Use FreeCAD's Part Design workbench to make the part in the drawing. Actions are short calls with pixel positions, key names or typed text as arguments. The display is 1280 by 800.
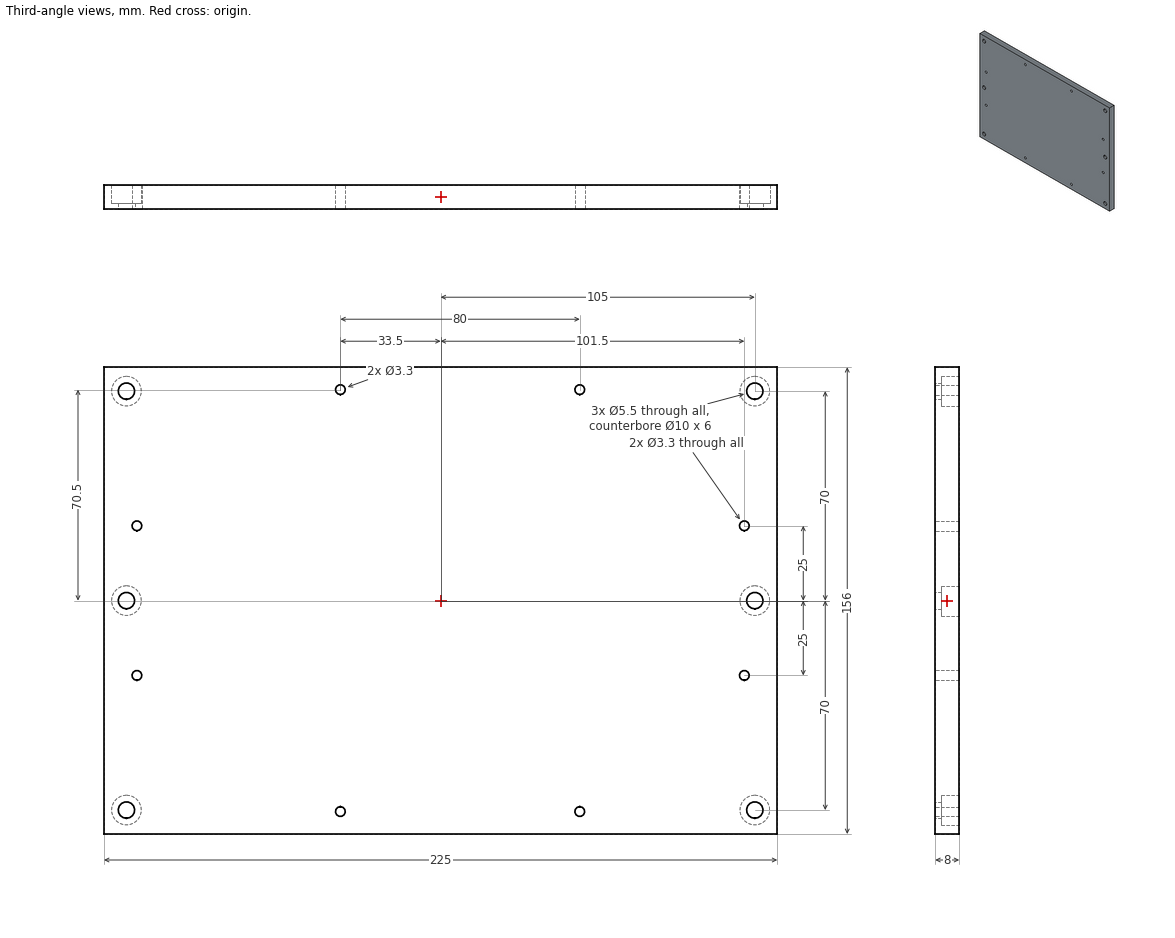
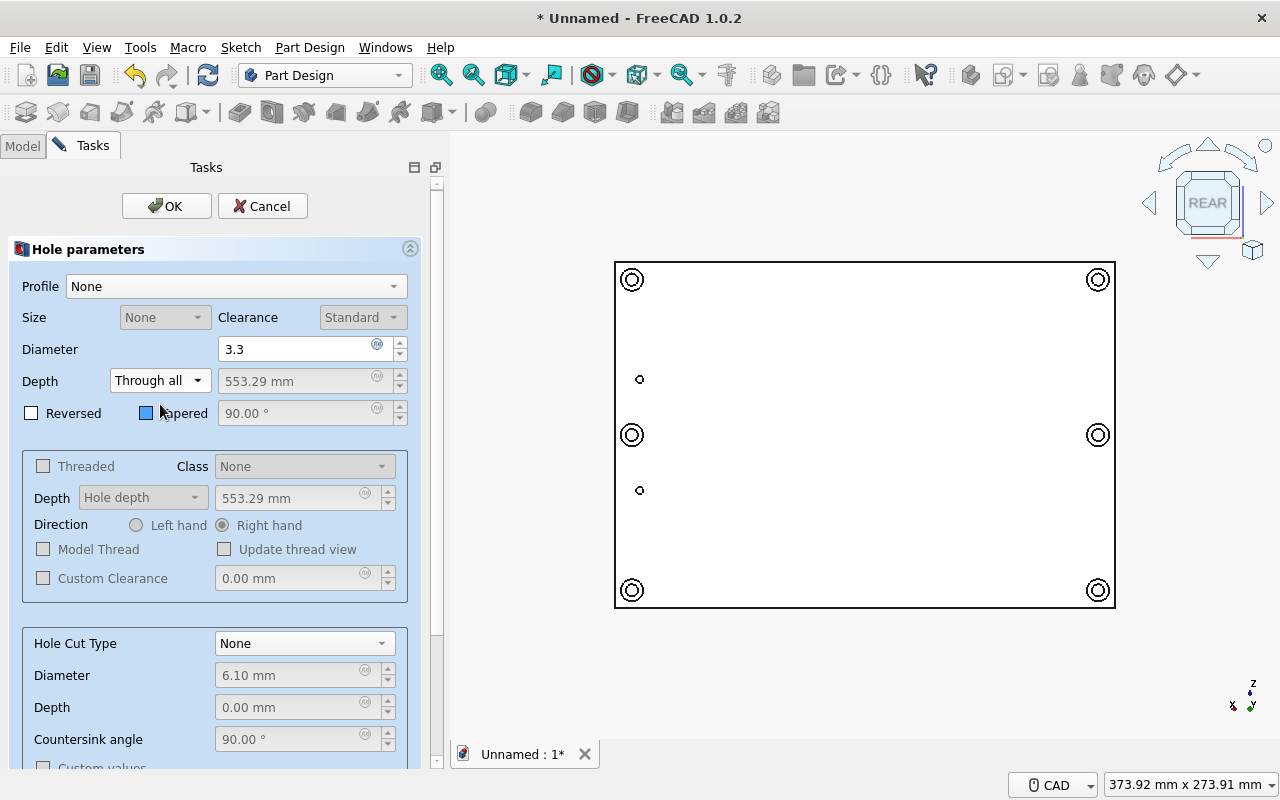
click(167, 206)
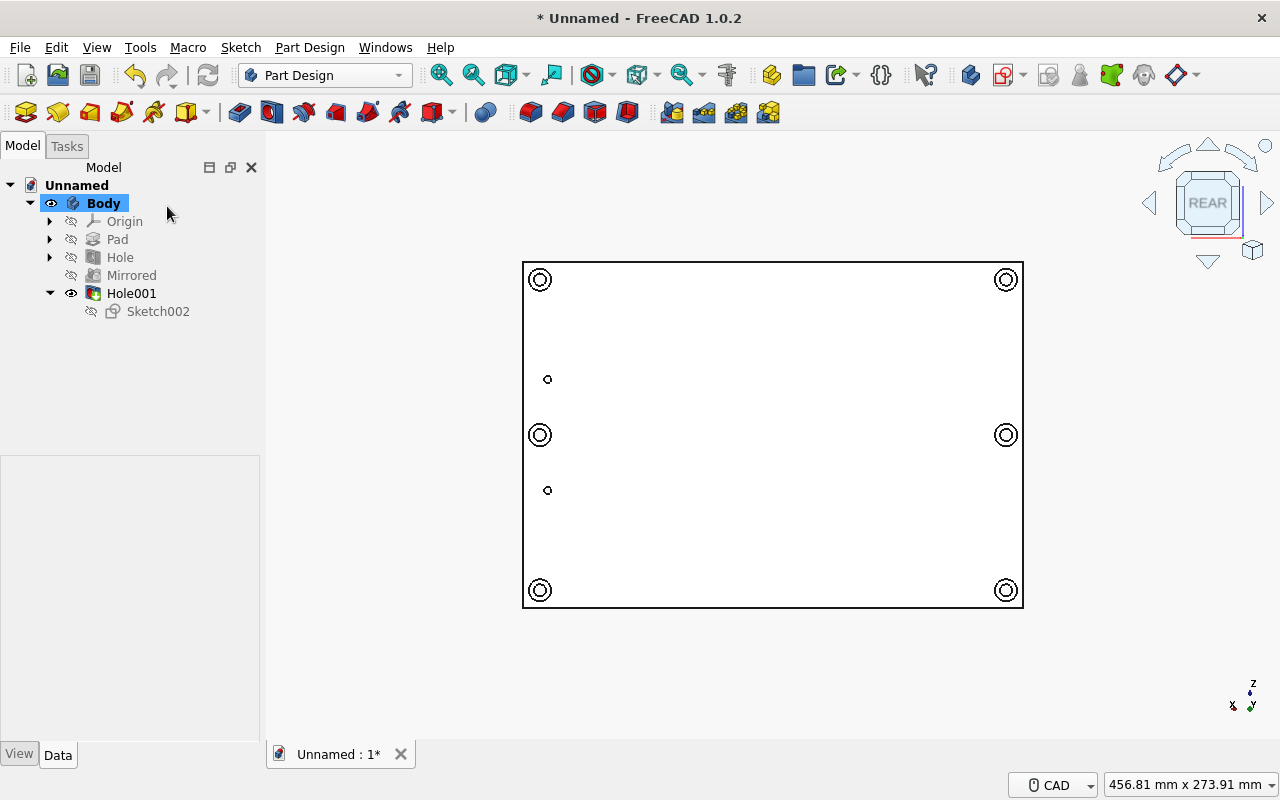
click(773, 434)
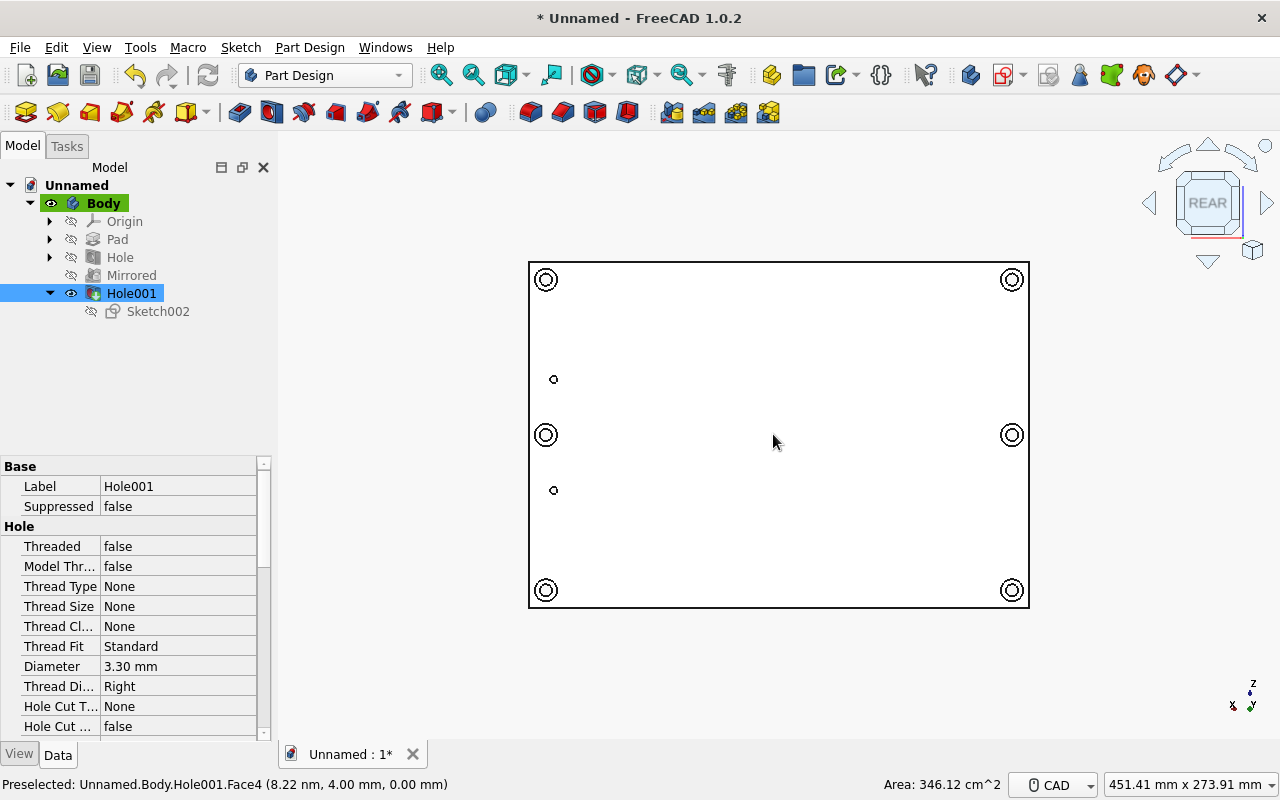
click(1004, 76)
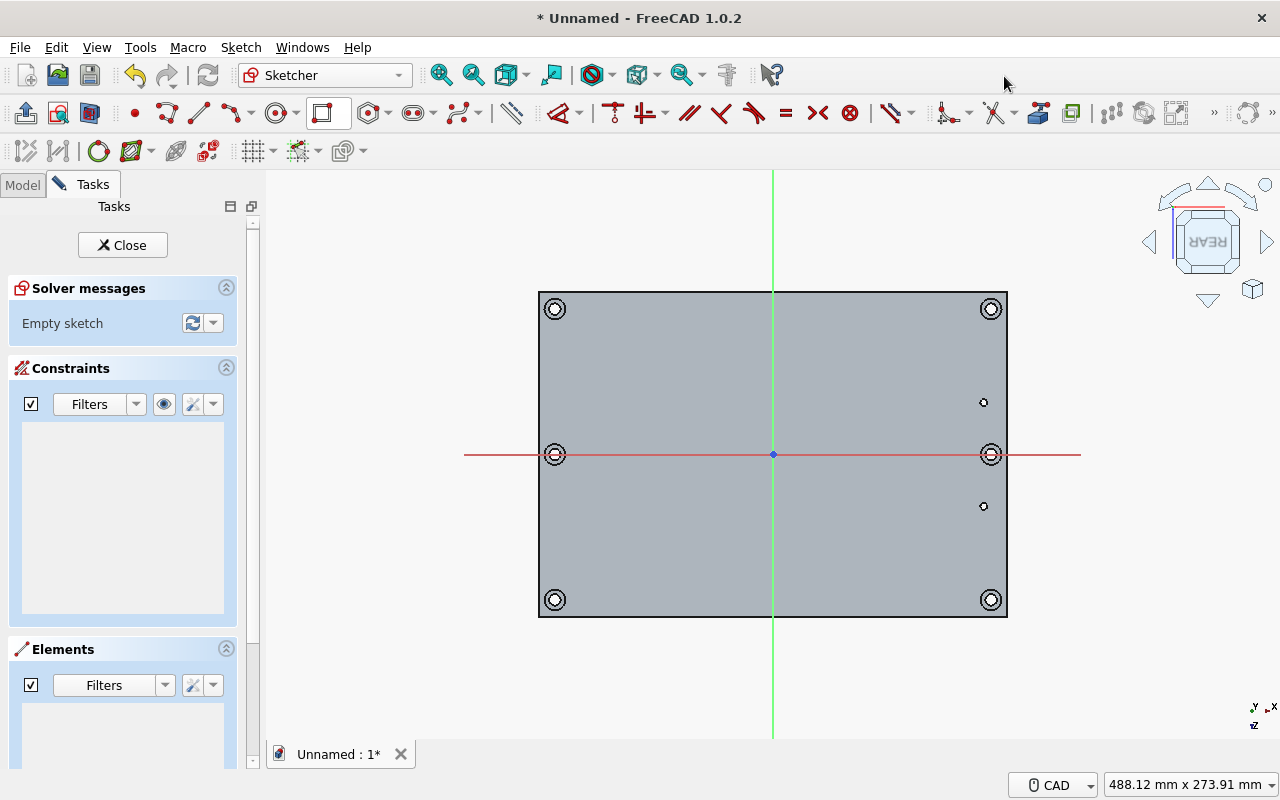
scroll(853, 591, up, 4)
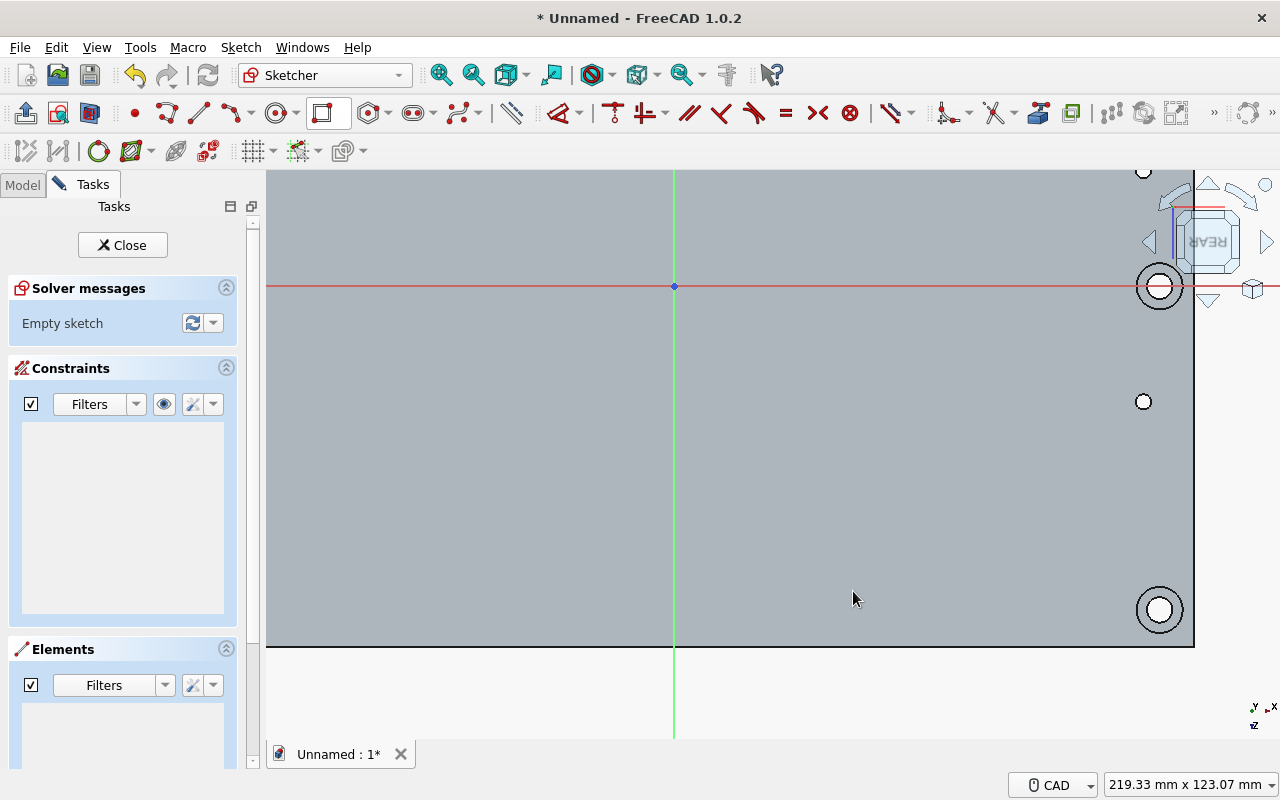
click(276, 114)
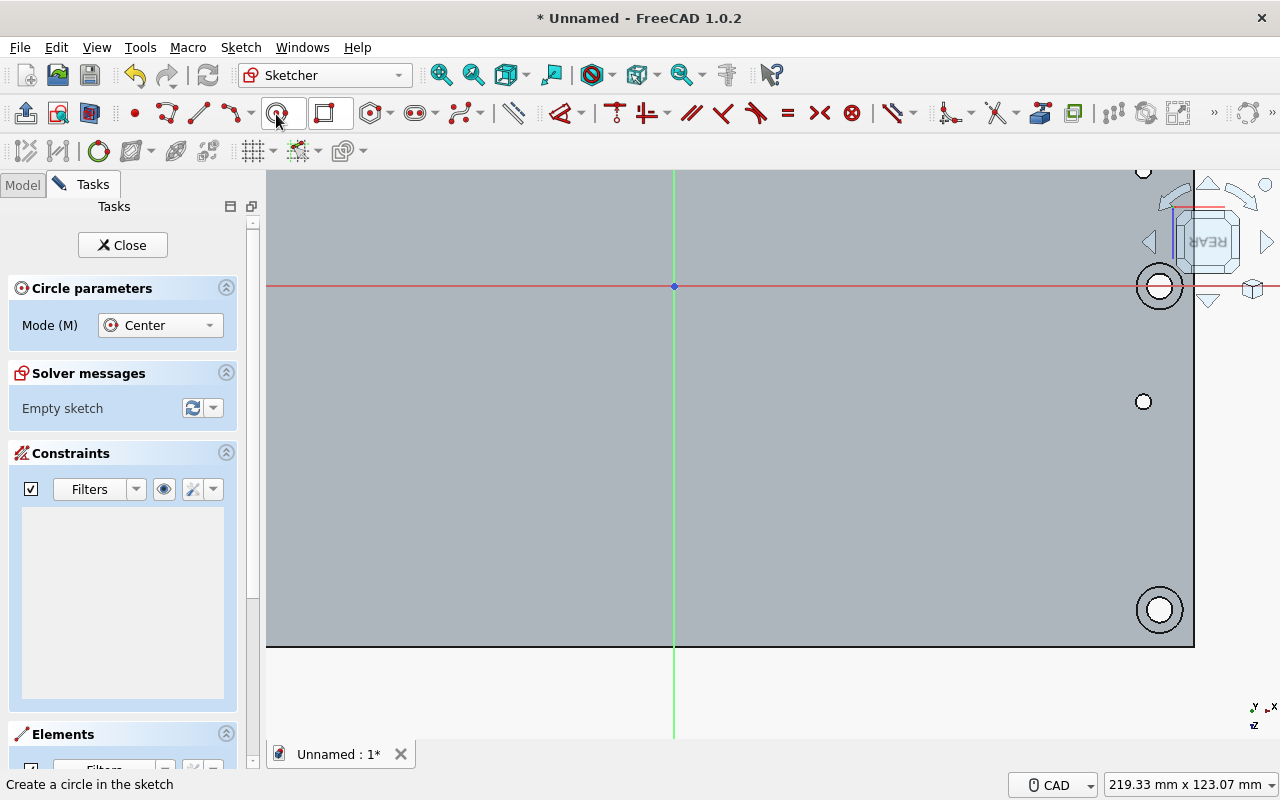
scroll(519, 612, up, 6)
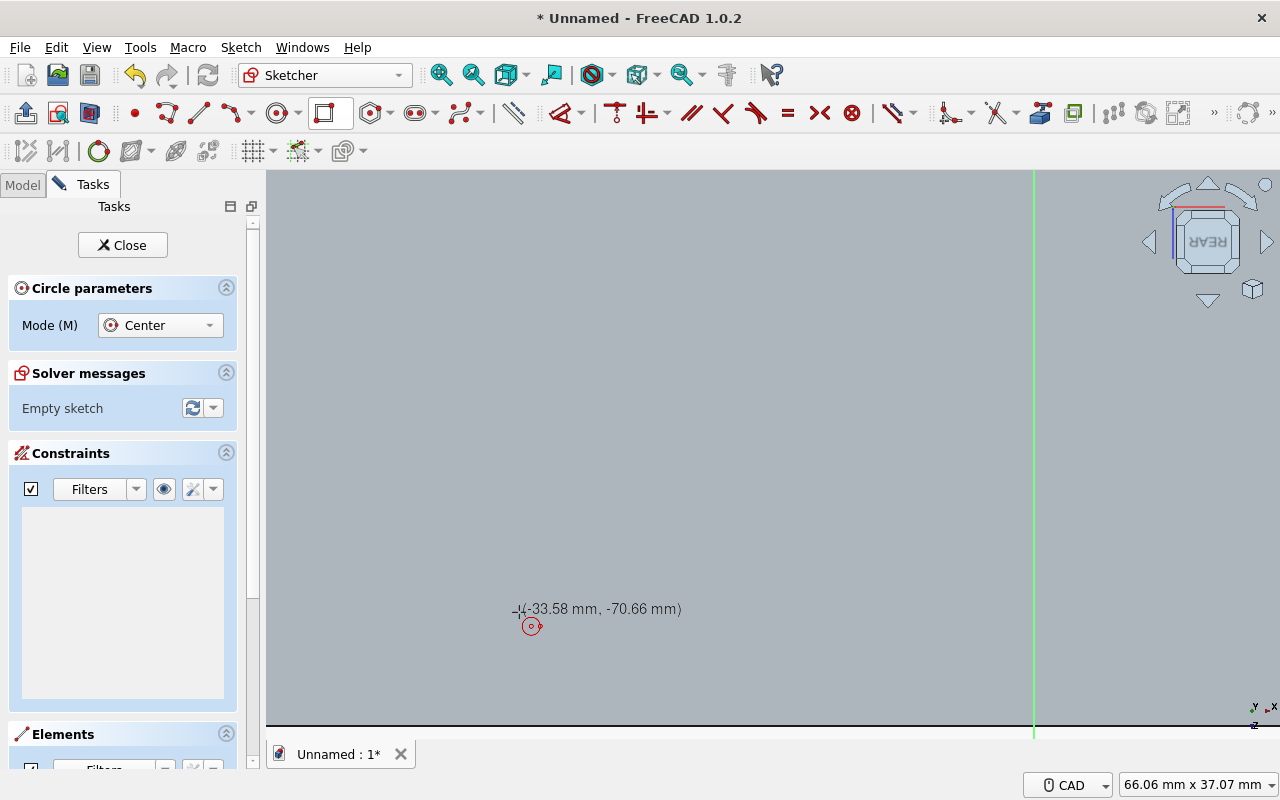
click(520, 611)
click(538, 593)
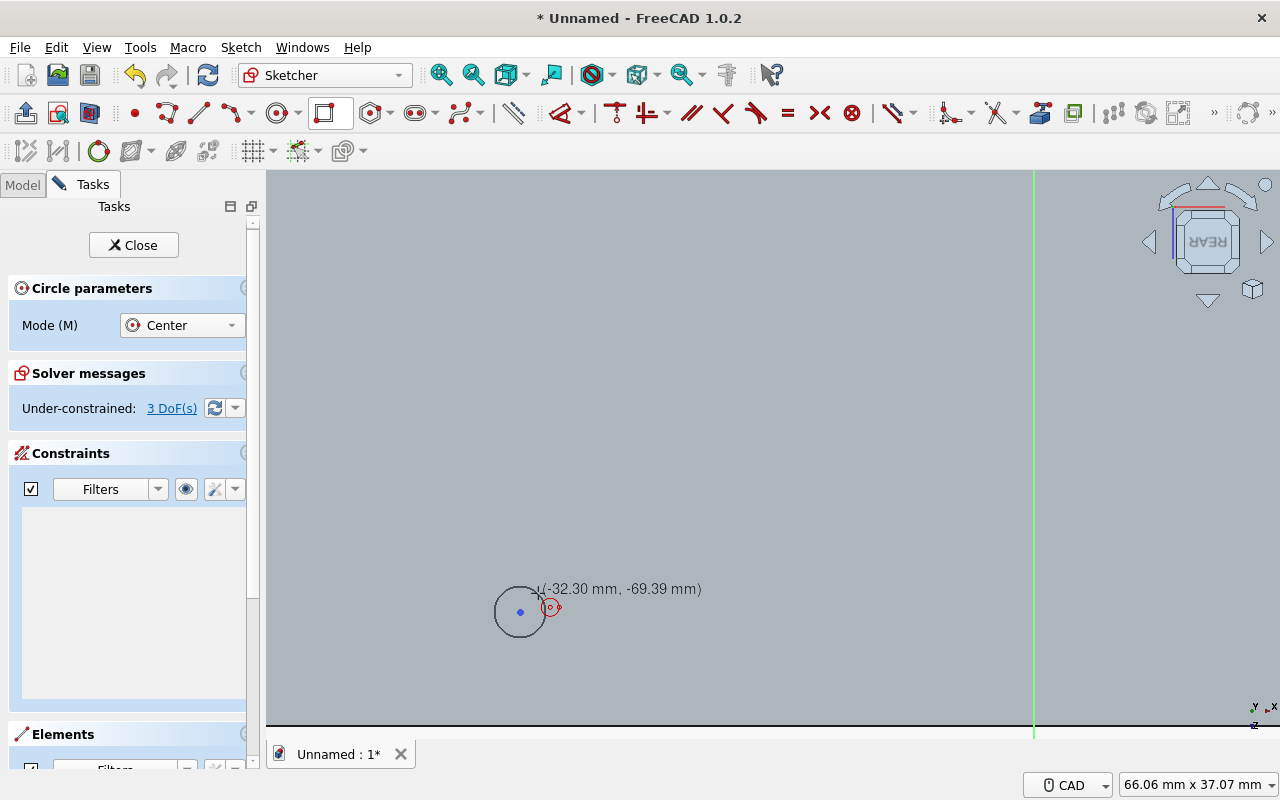
scroll(520, 615, down, 6)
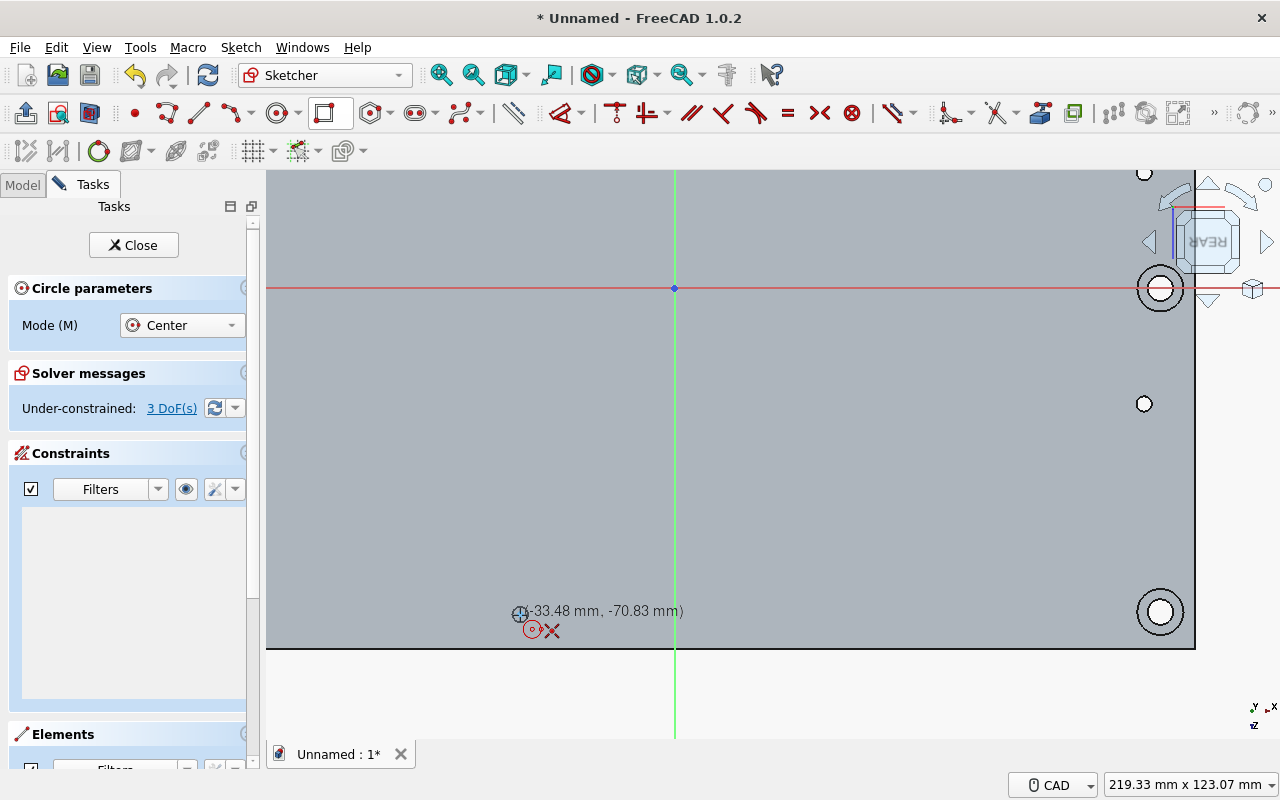
scroll(890, 614, up, 6)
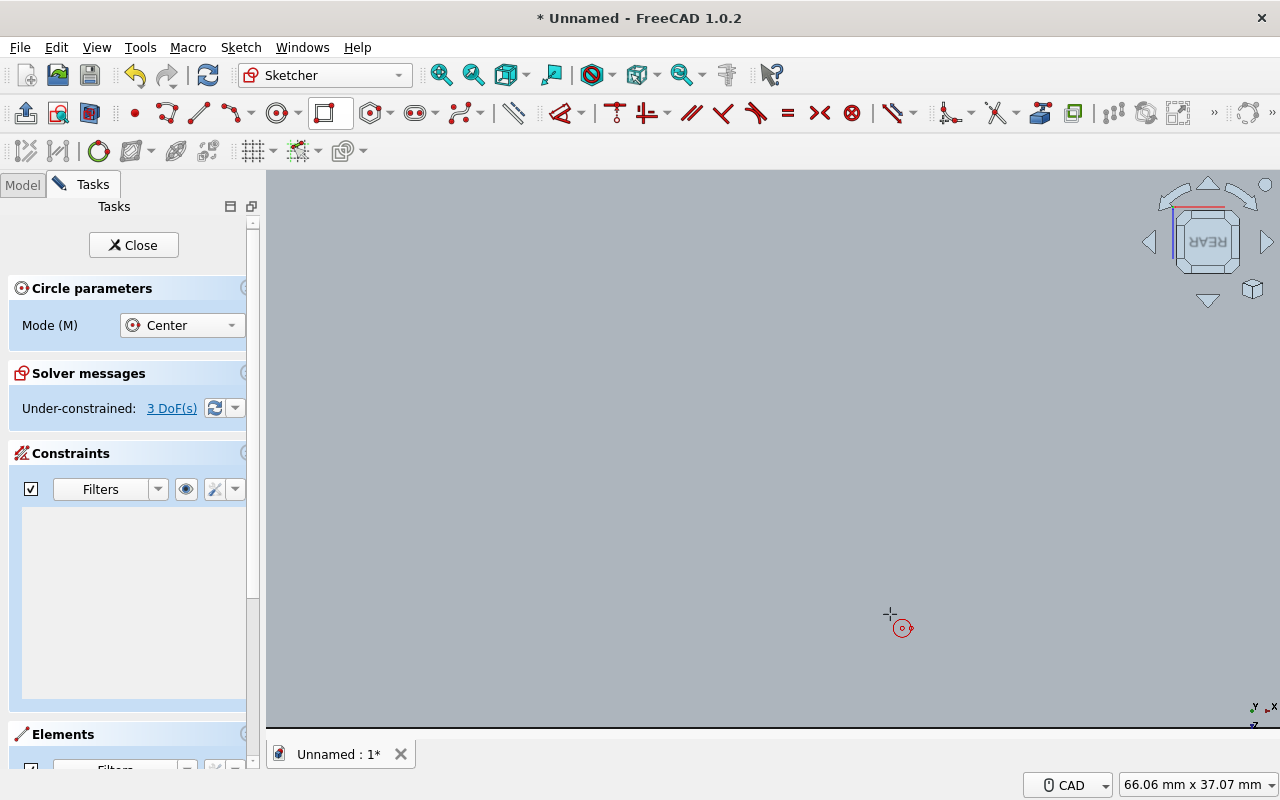
click(888, 613)
click(906, 595)
key(Escape)